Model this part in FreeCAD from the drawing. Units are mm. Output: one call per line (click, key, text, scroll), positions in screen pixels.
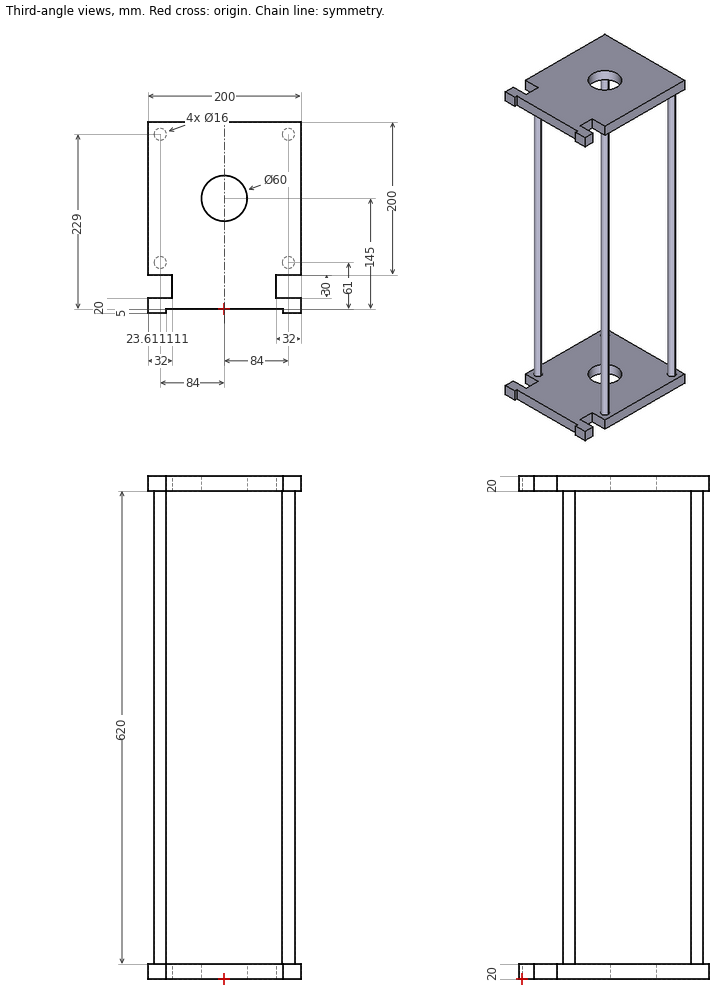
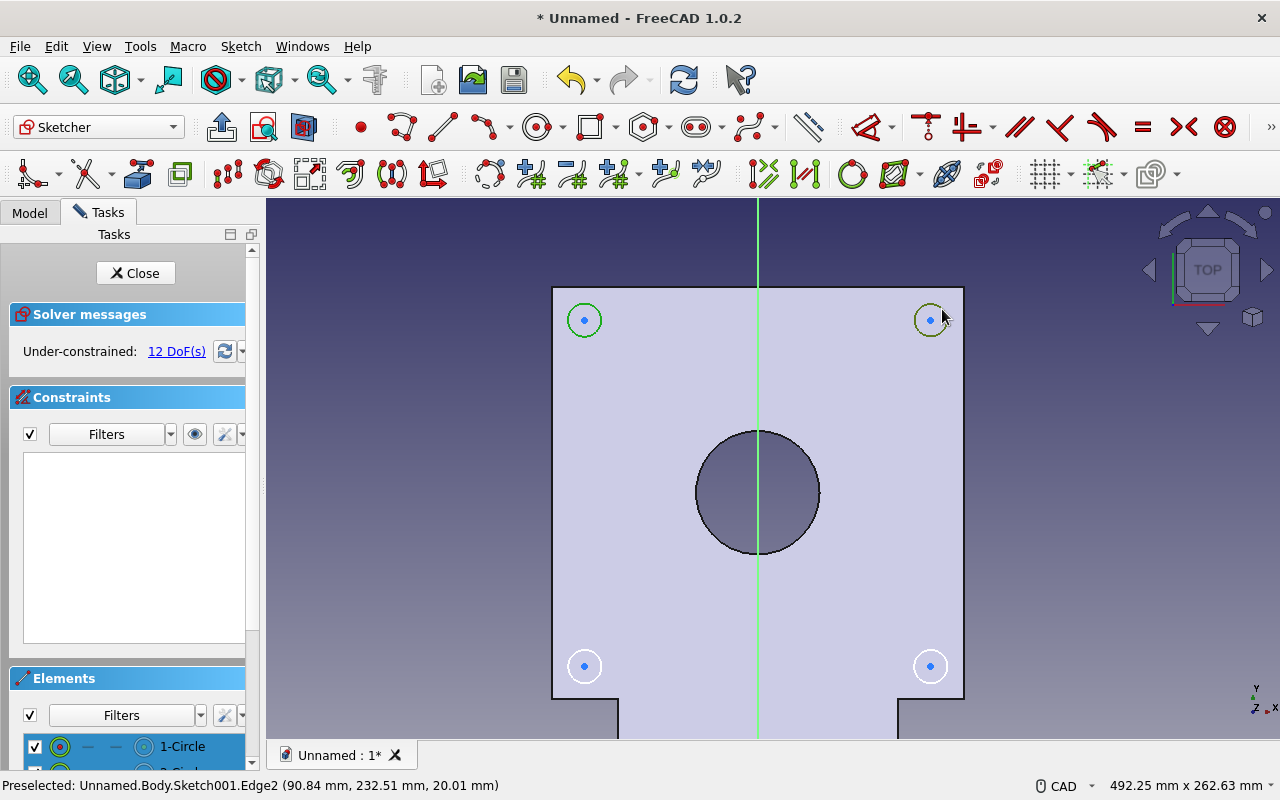
click(942, 655)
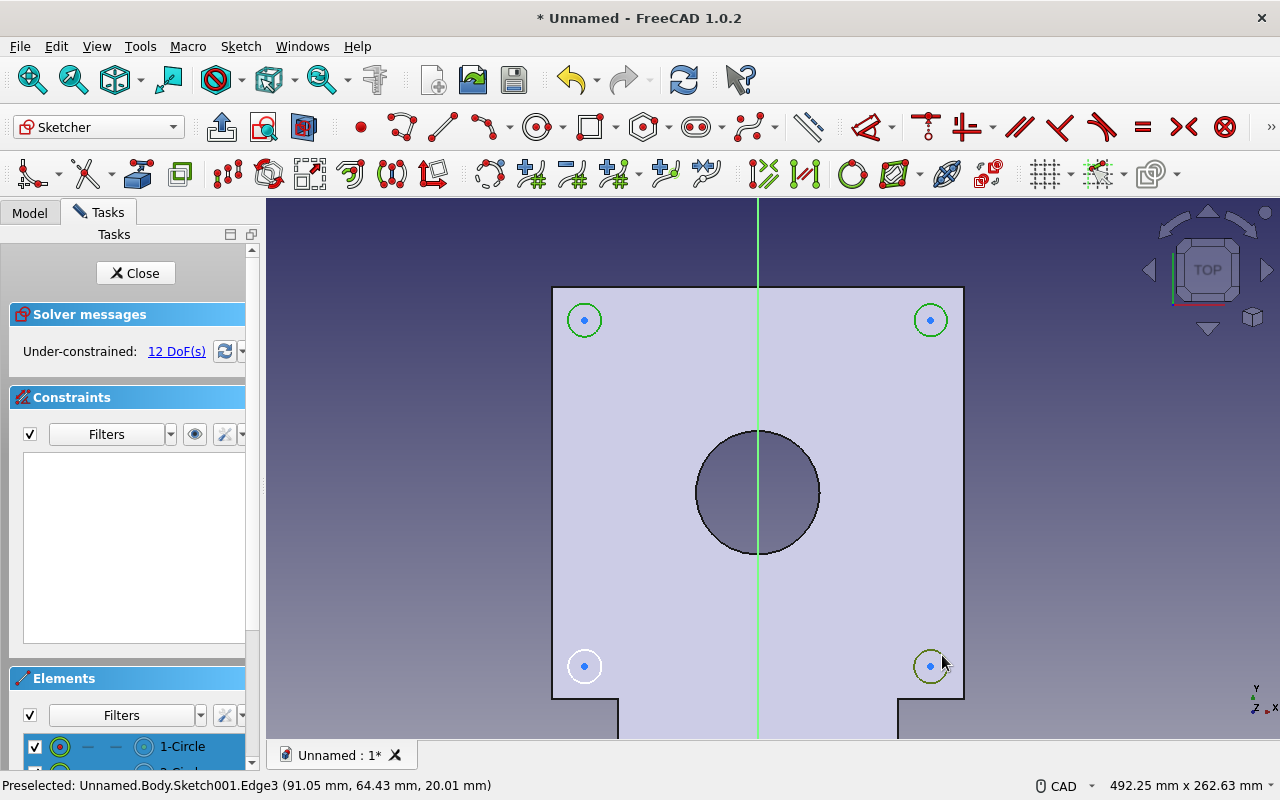
click(597, 655)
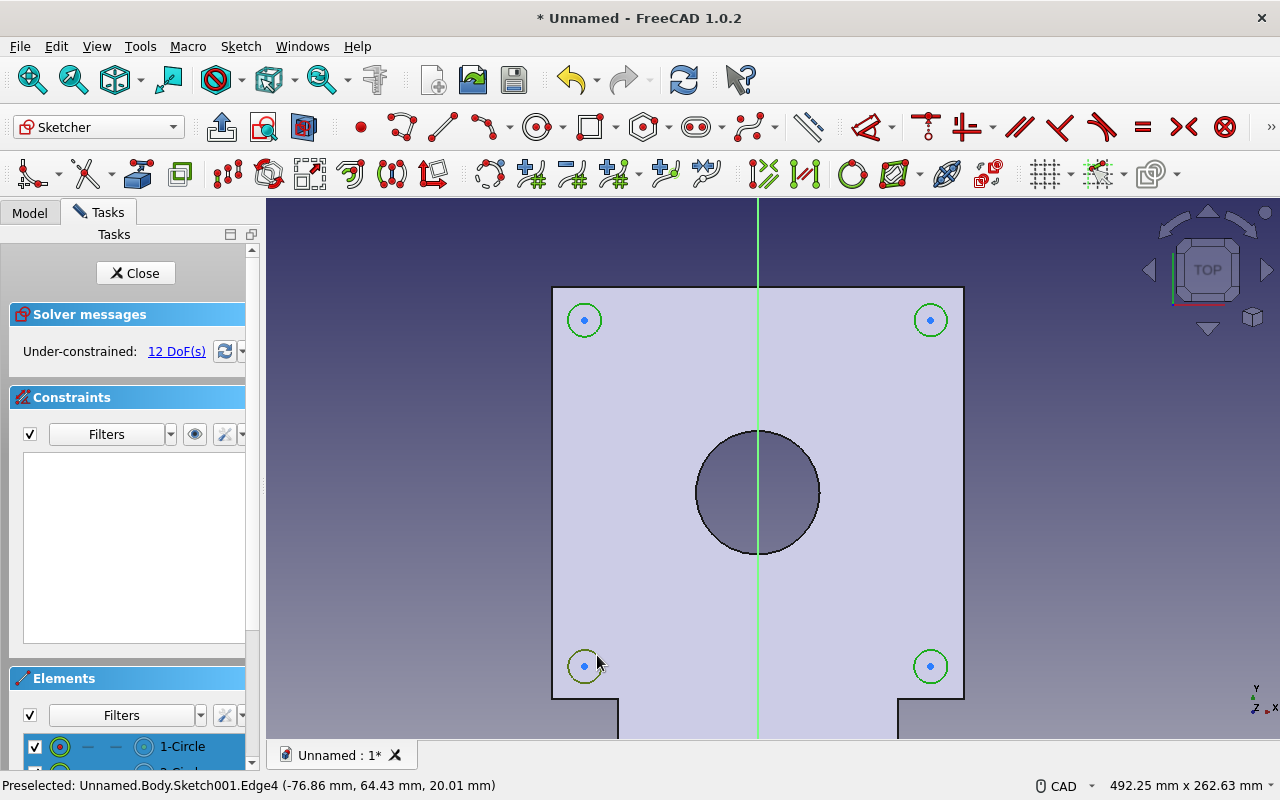
click(1143, 128)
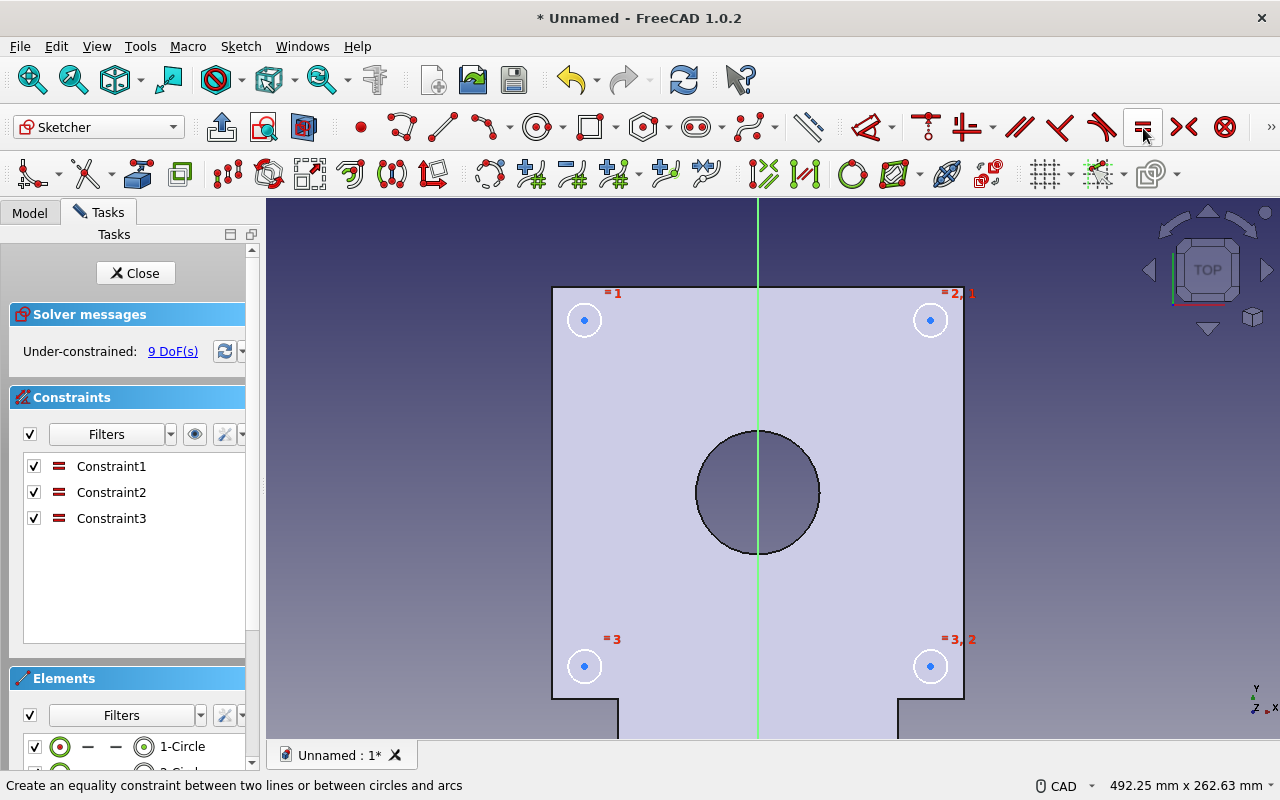
click(585, 320)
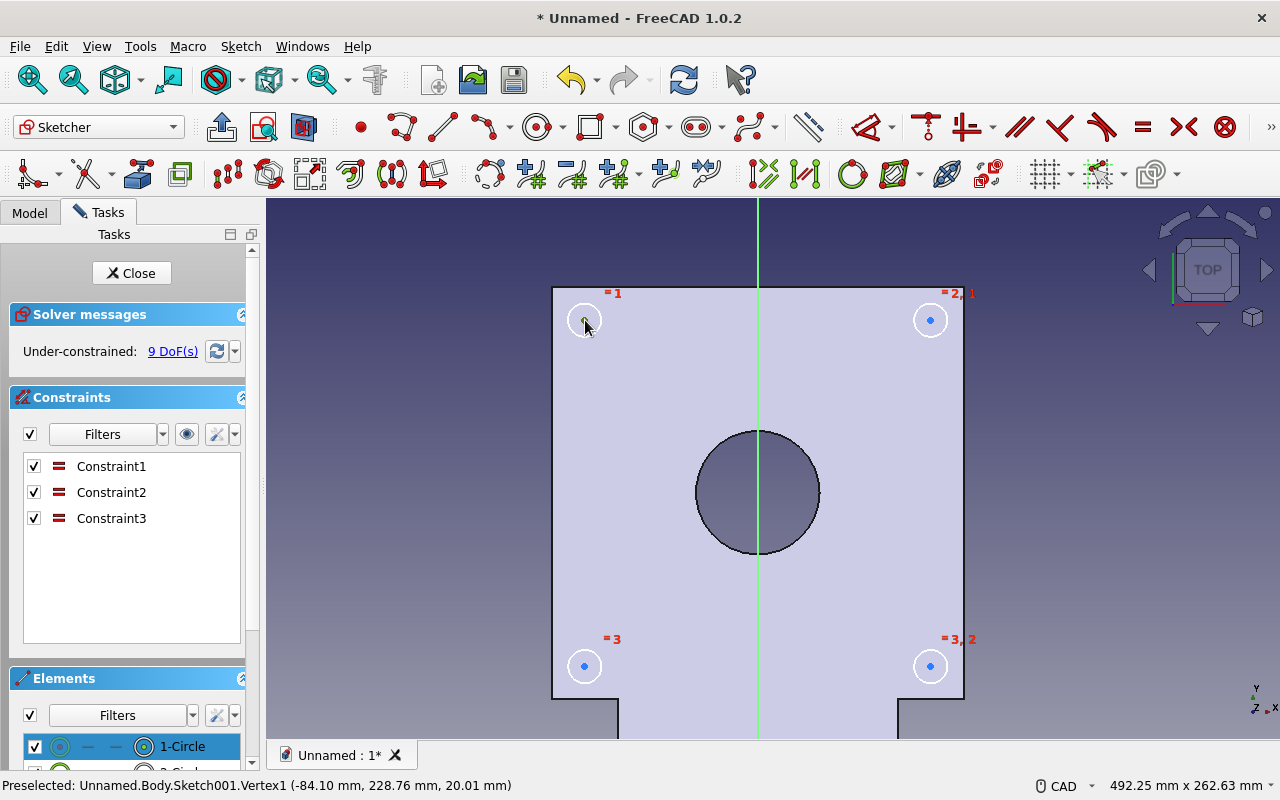
click(931, 320)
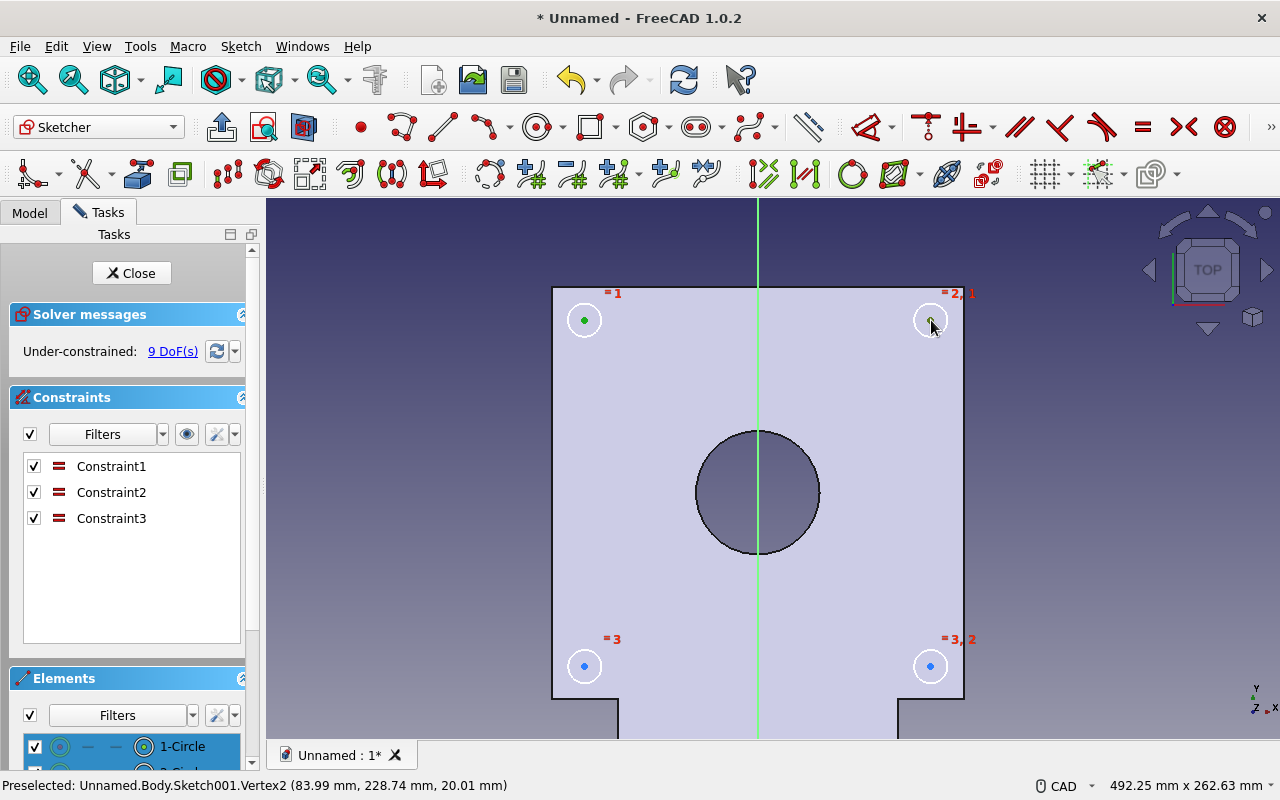
click(992, 128)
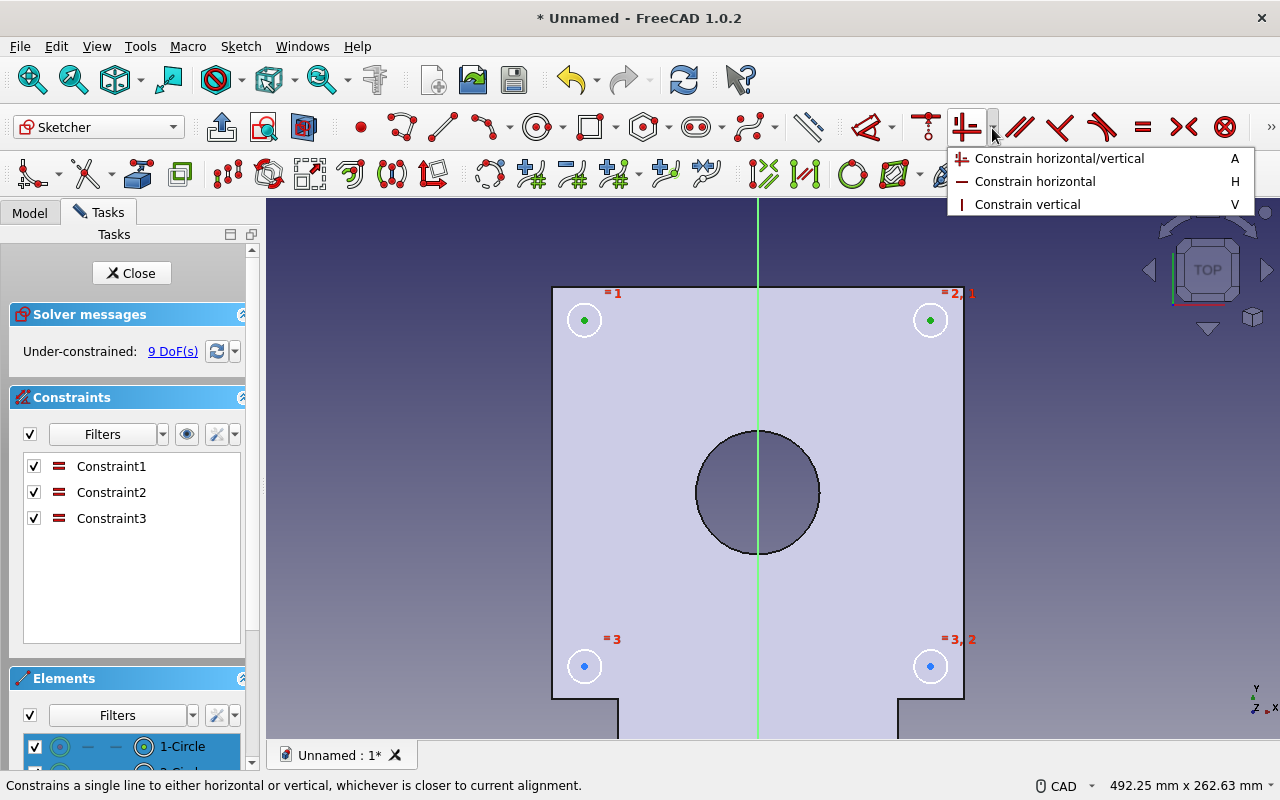
click(1101, 182)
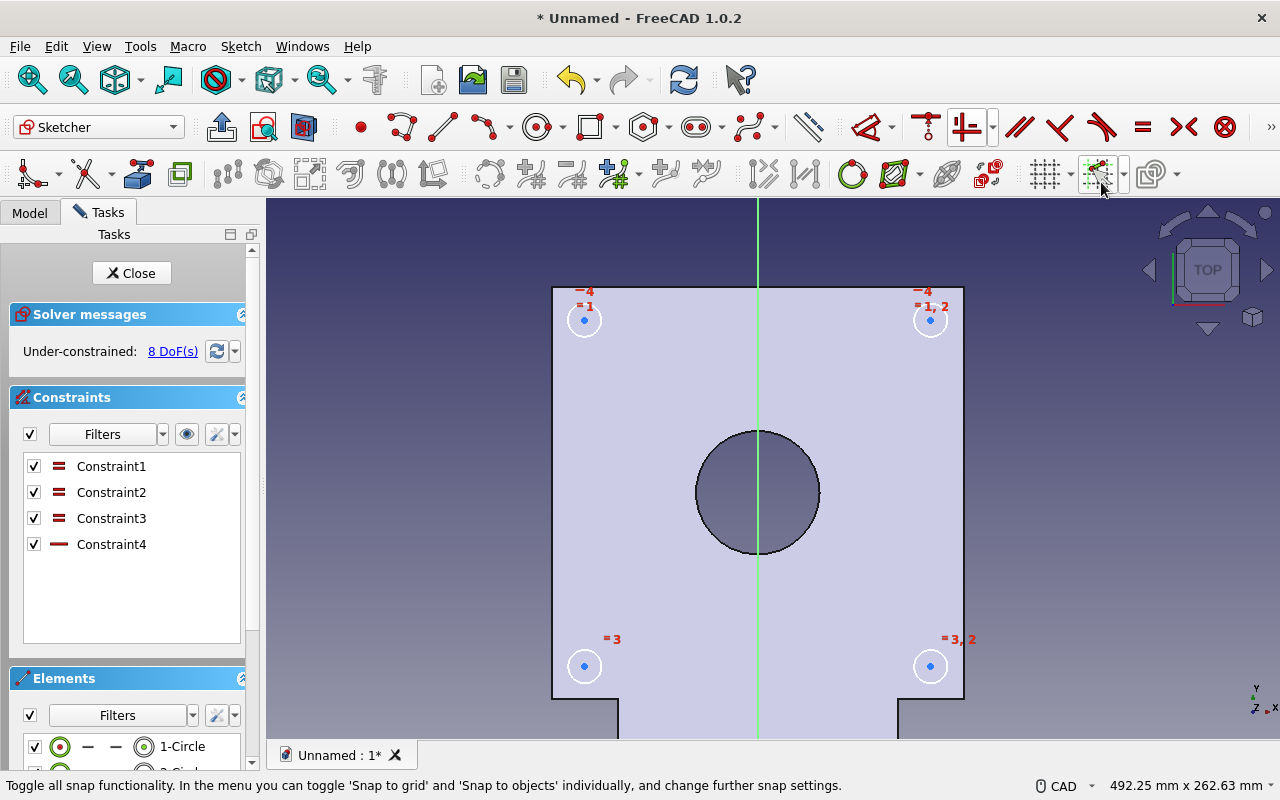
click(931, 320)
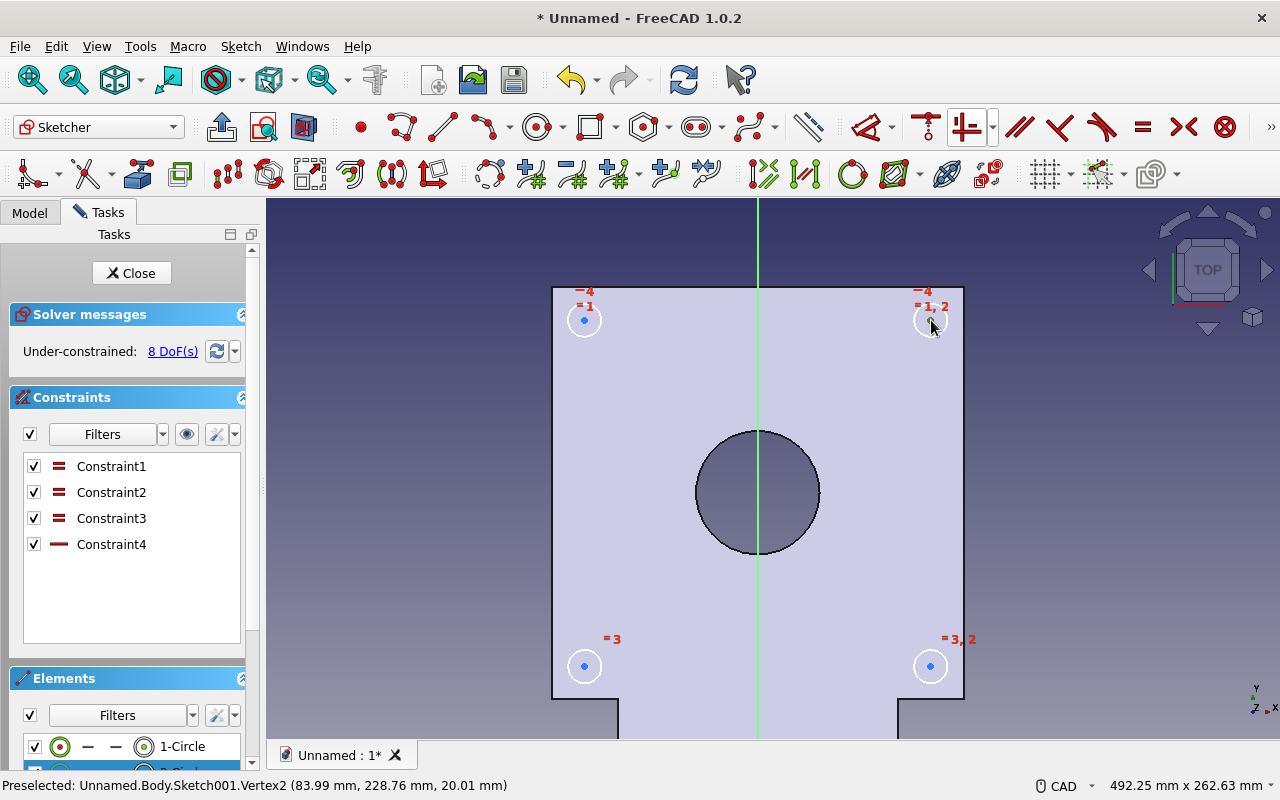
click(931, 667)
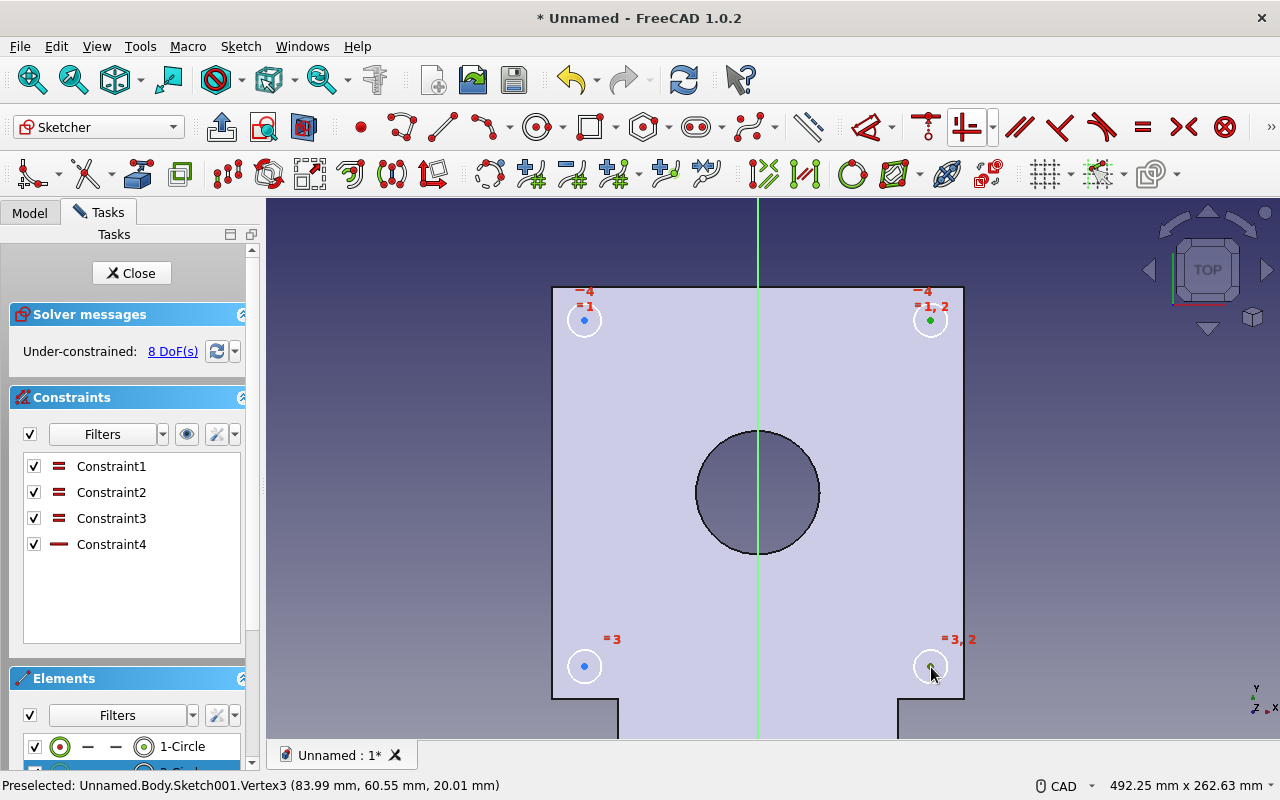
key(v)